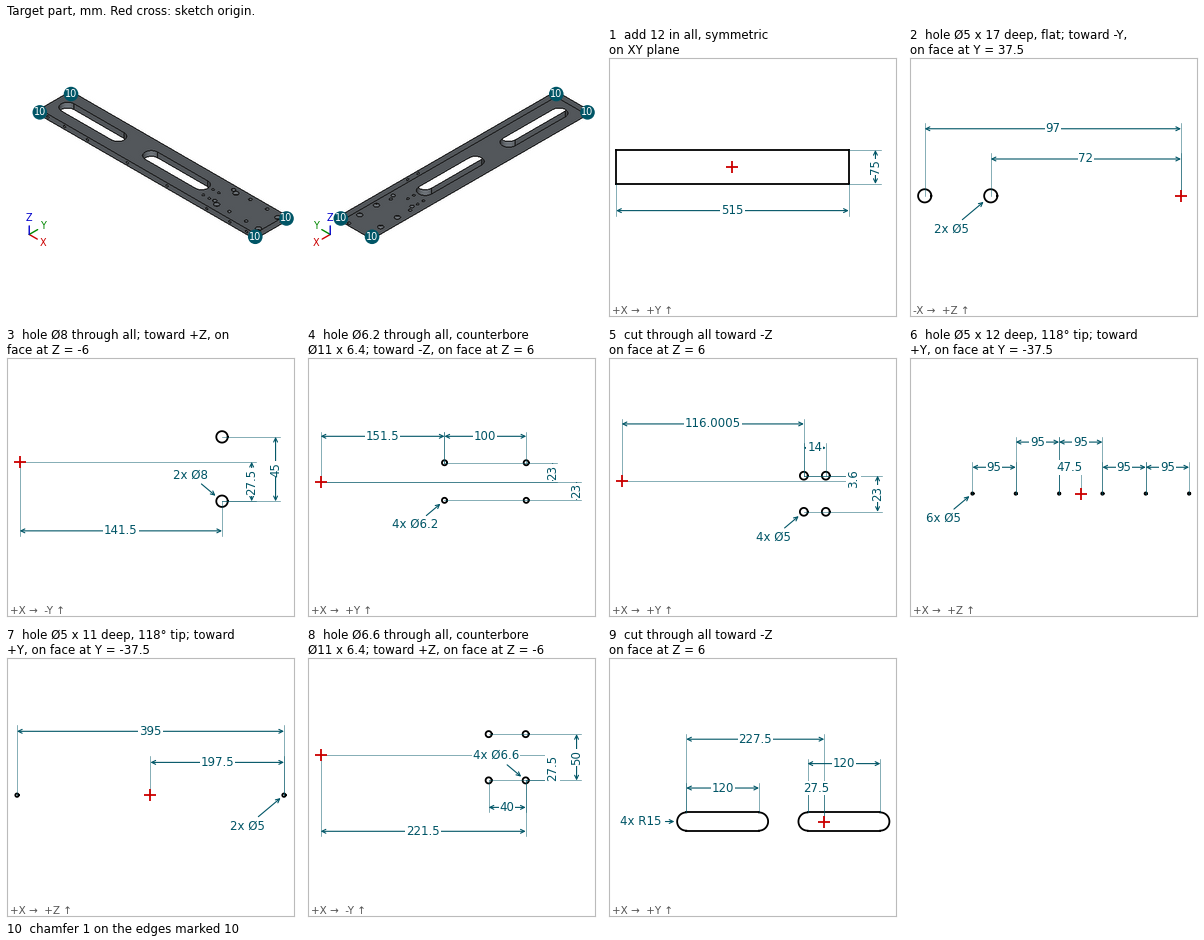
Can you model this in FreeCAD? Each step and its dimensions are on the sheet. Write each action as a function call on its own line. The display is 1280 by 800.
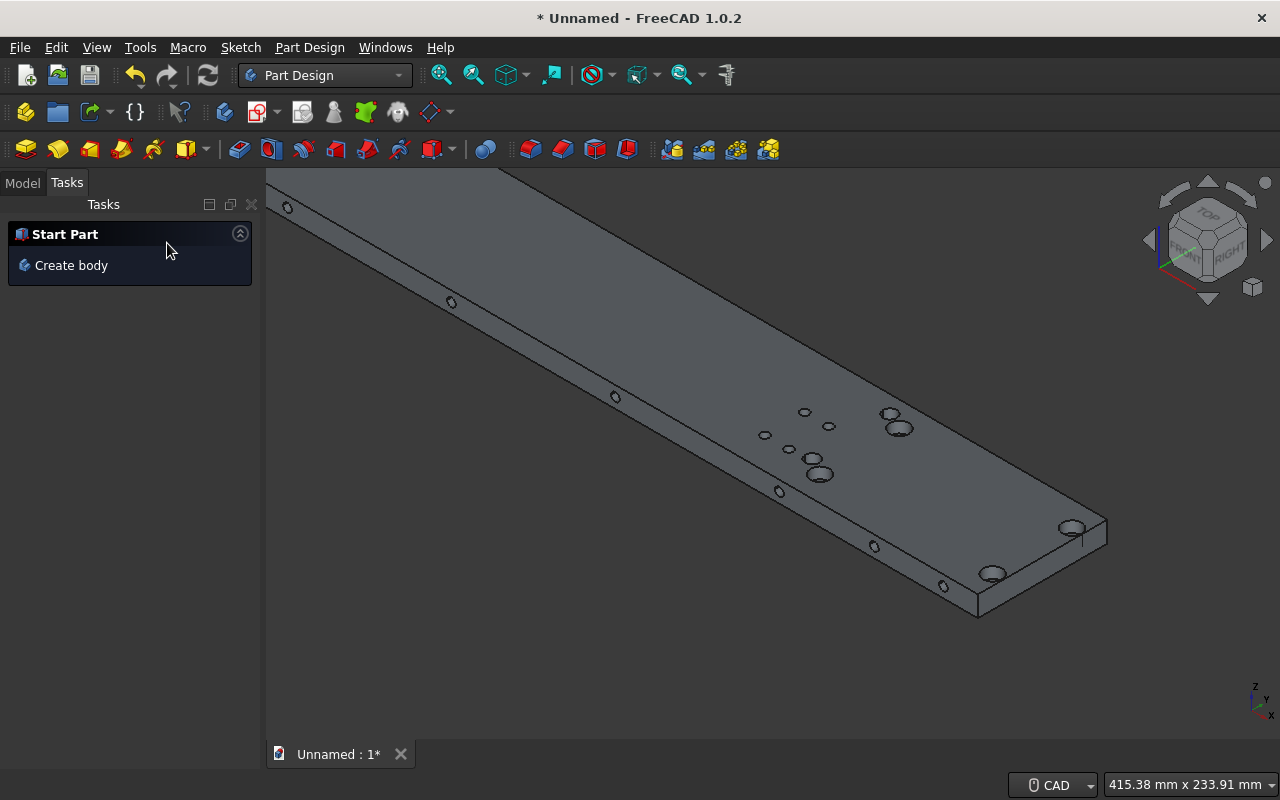
key(v)
key(f)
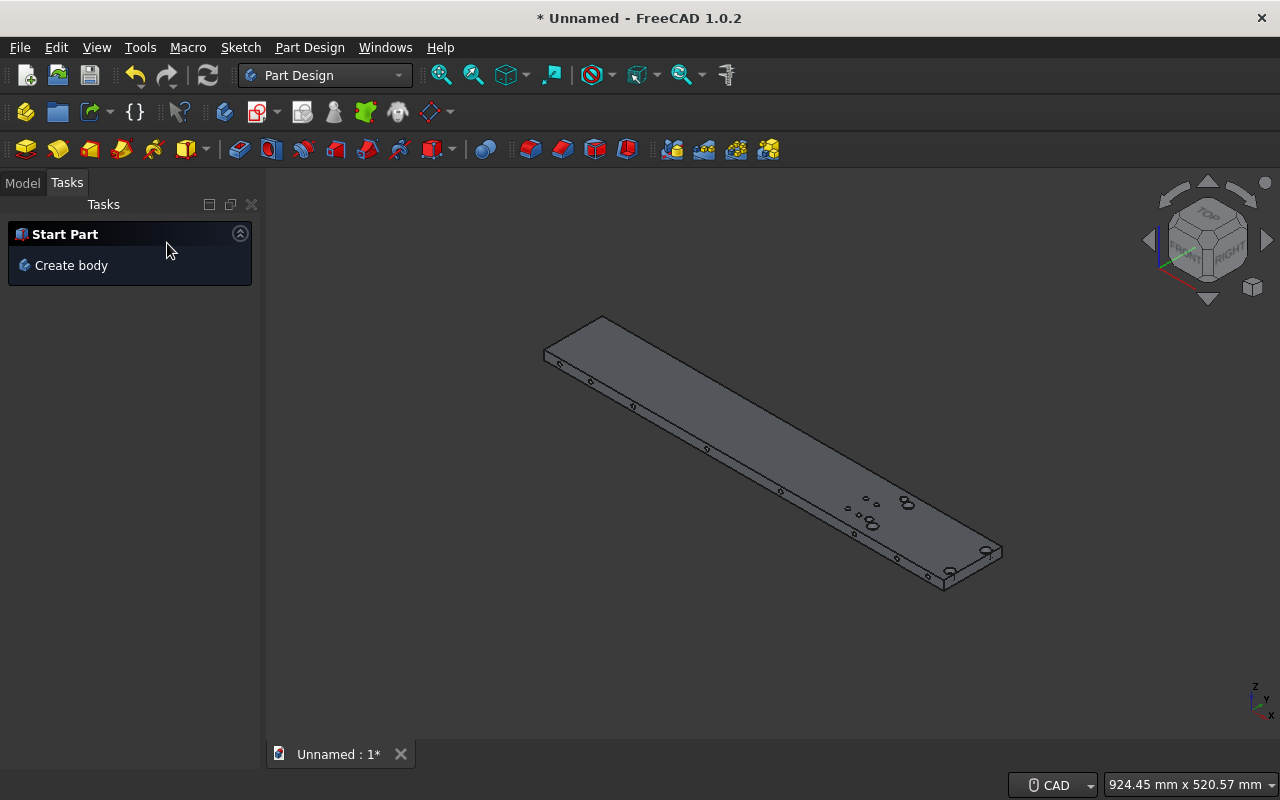
key(5)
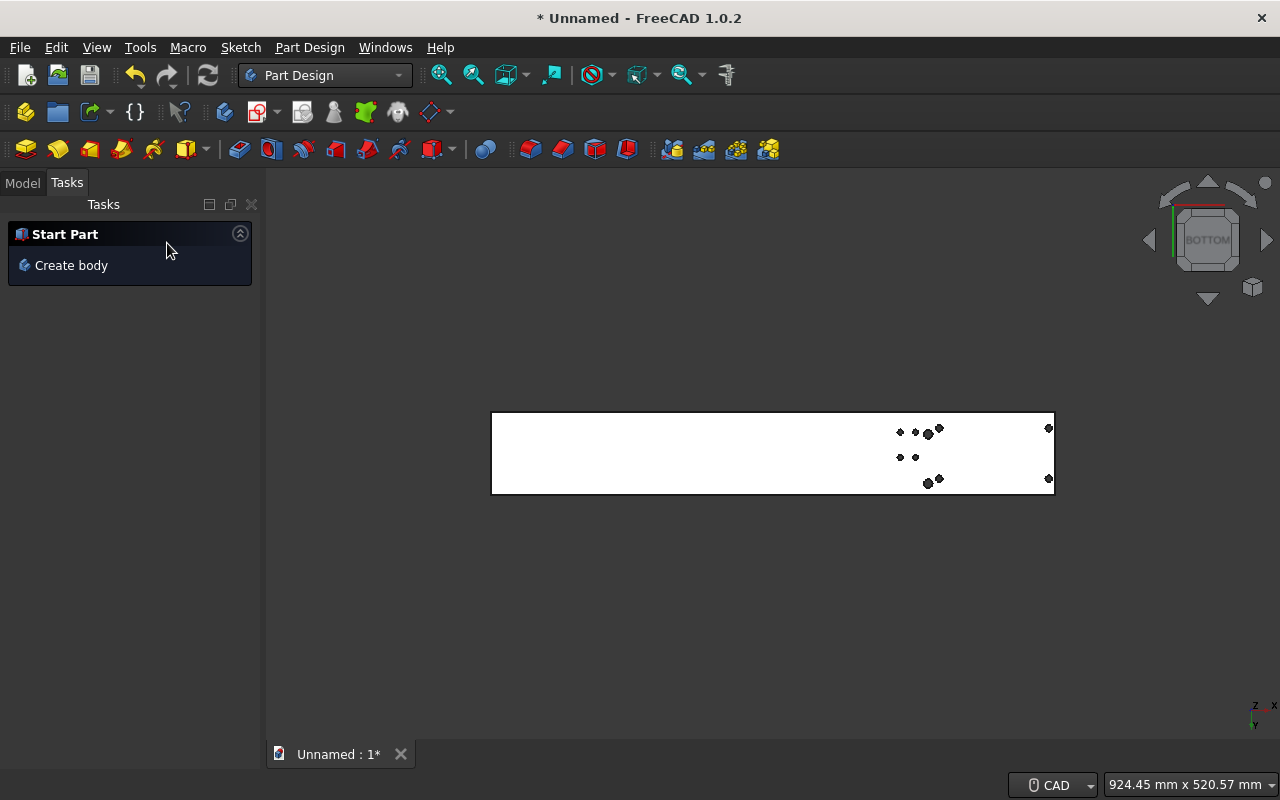
click(854, 452)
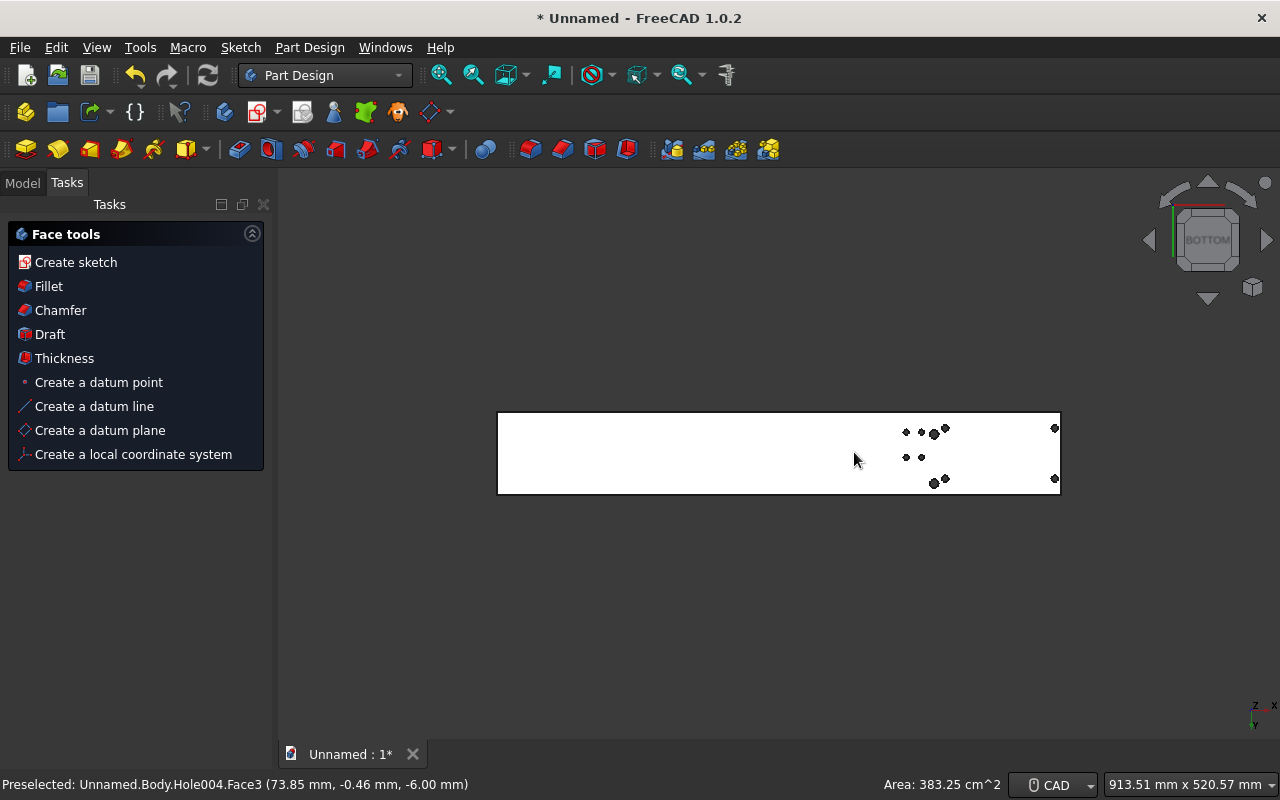
click(258, 112)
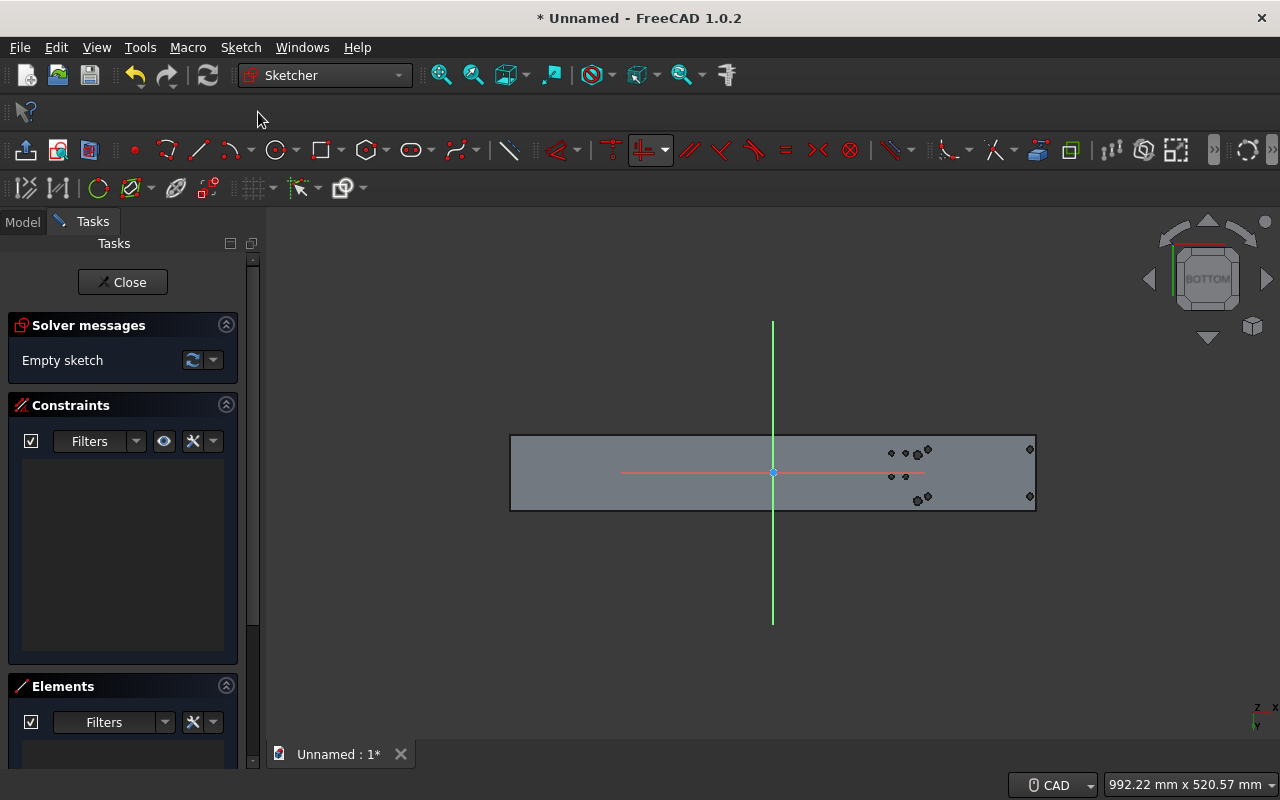
scroll(1033, 476, up, 9)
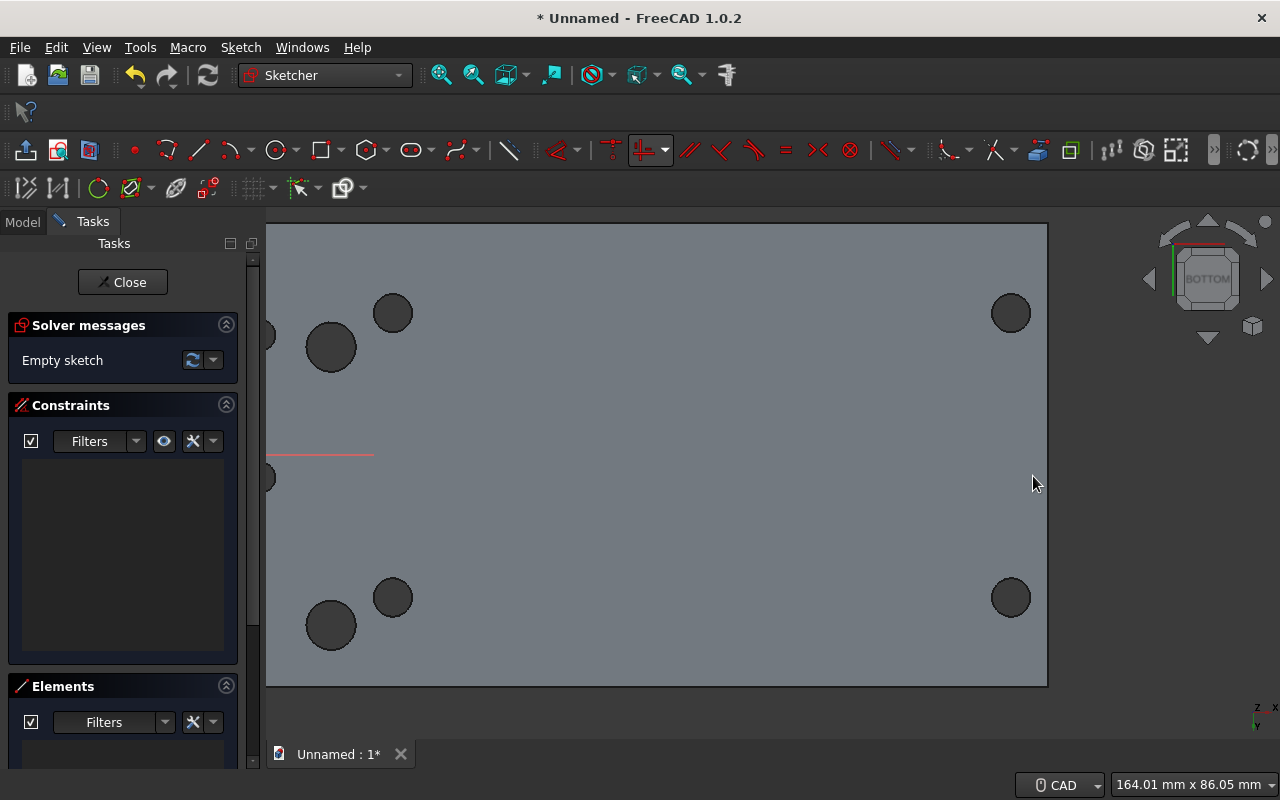
key(g)
key(c)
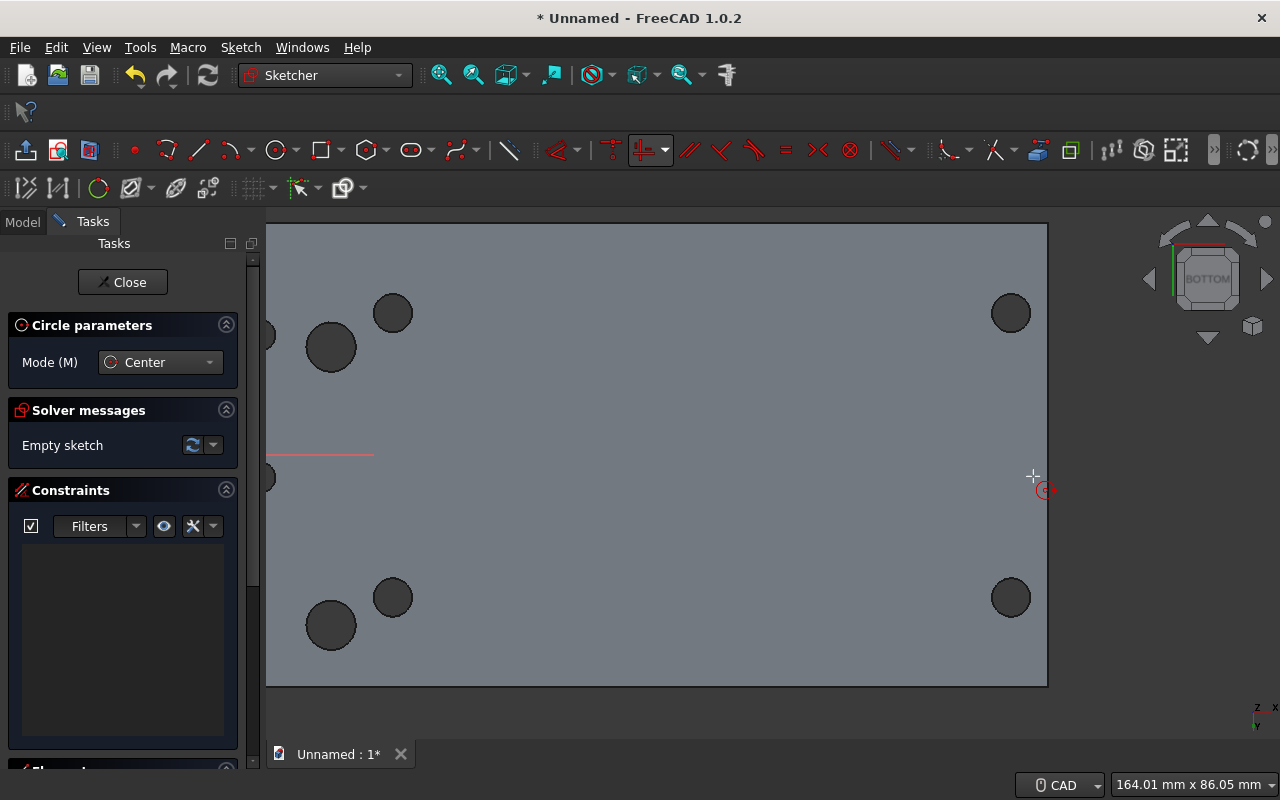
click(826, 625)
click(840, 611)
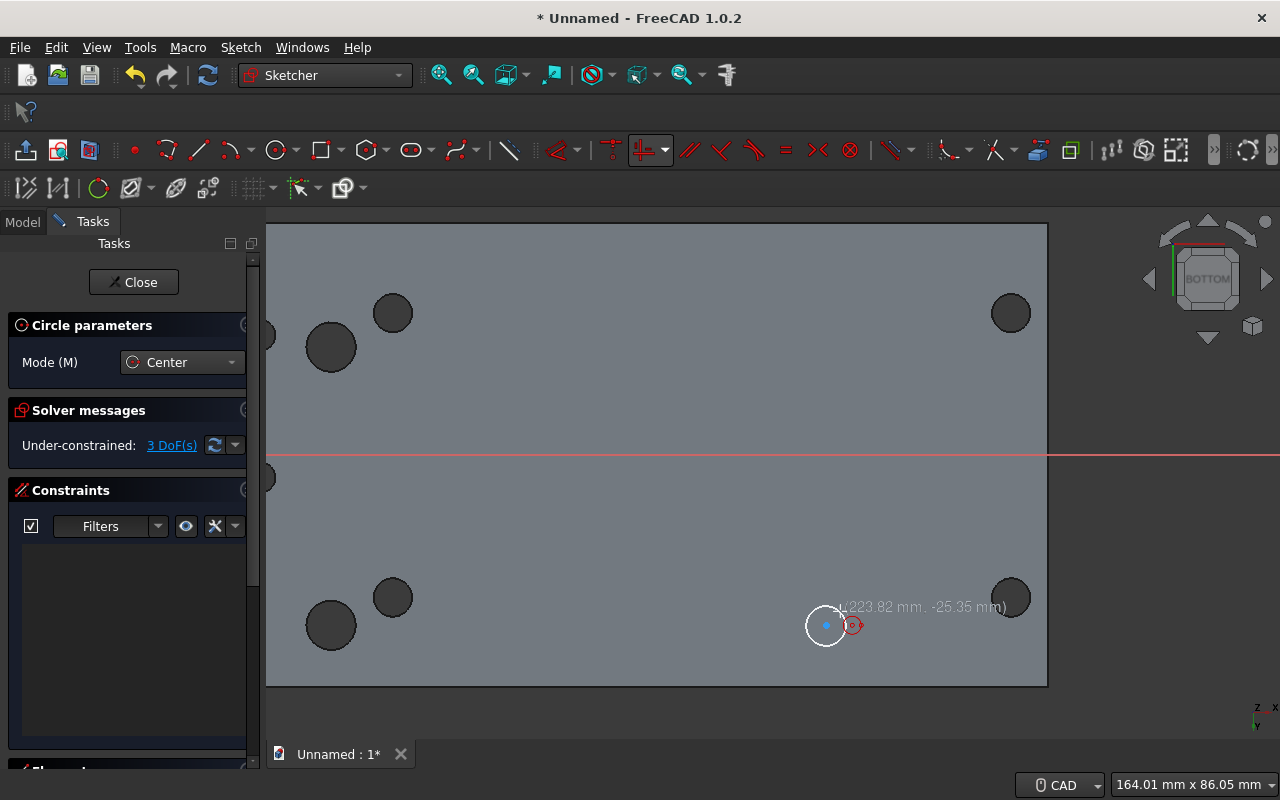
click(578, 625)
click(593, 611)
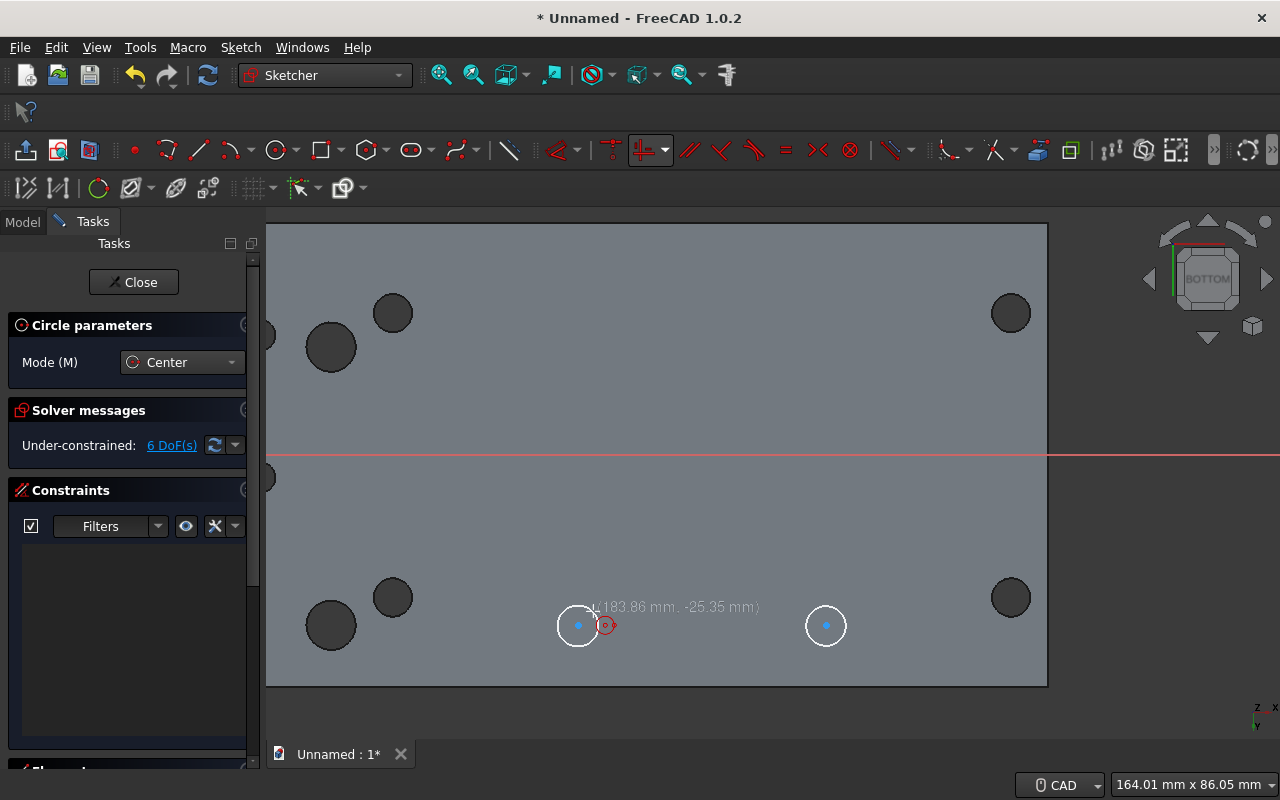
click(578, 316)
click(593, 302)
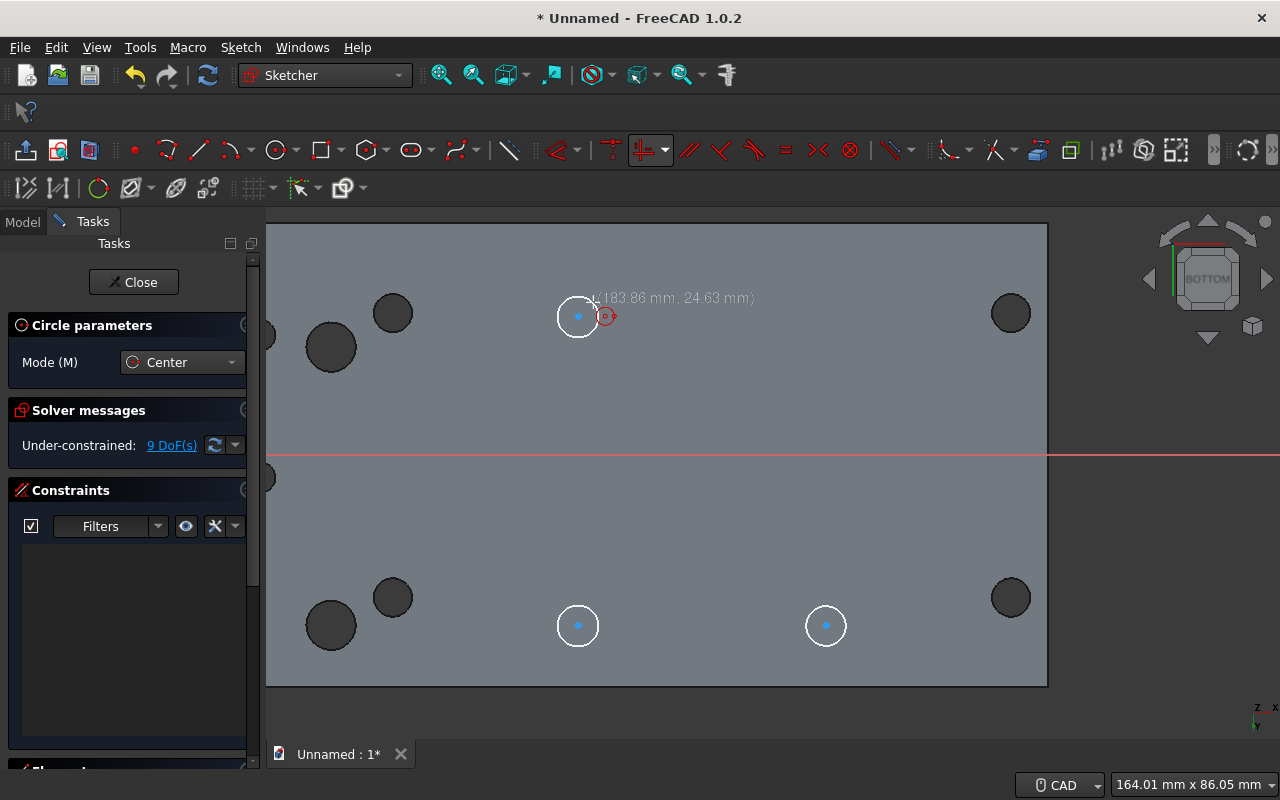
click(826, 316)
click(840, 302)
key(Escape)